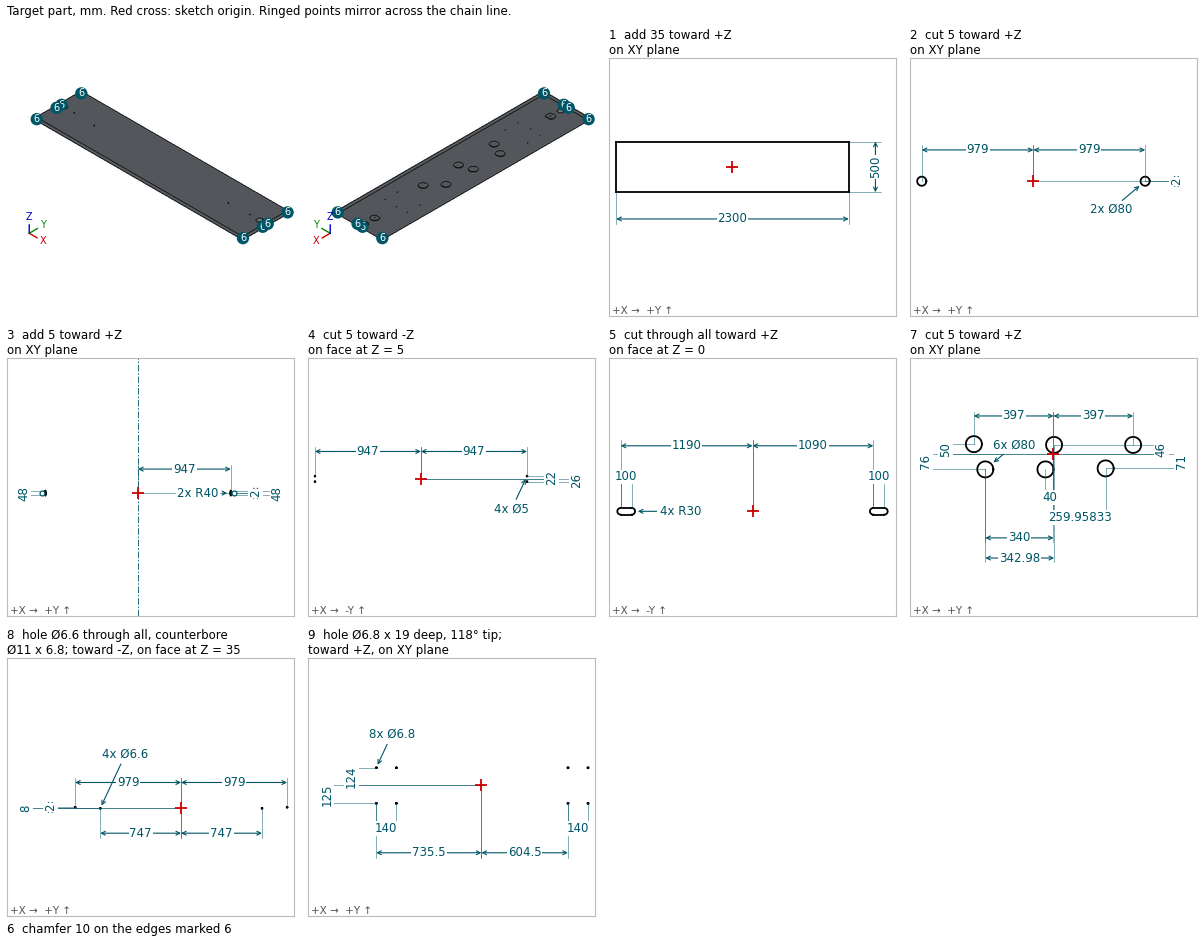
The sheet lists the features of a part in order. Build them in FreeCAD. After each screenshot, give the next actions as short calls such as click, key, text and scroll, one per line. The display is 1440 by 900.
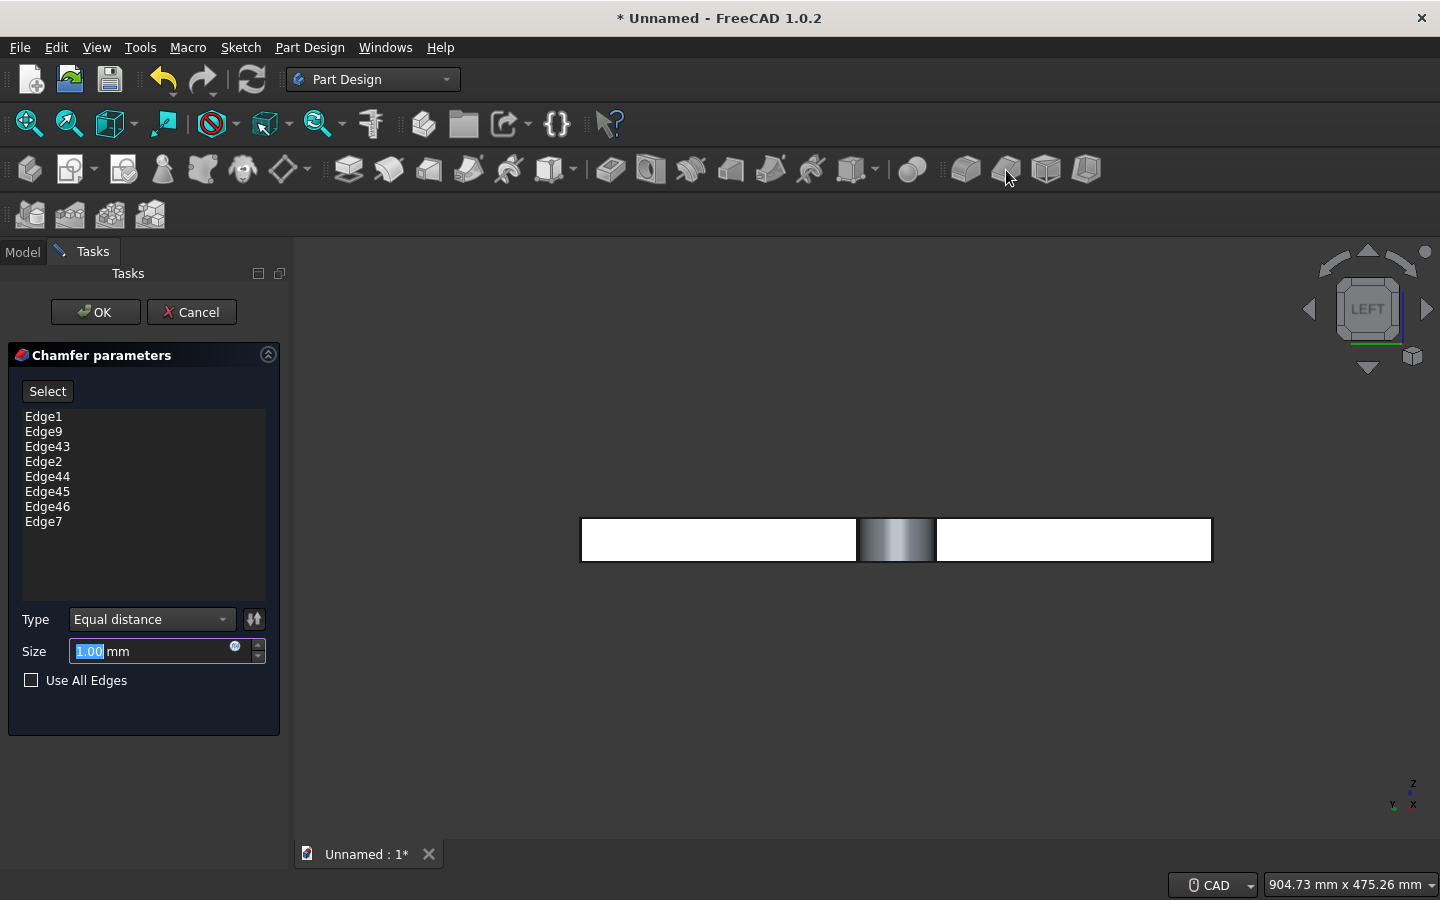
text(10)
key(Tab)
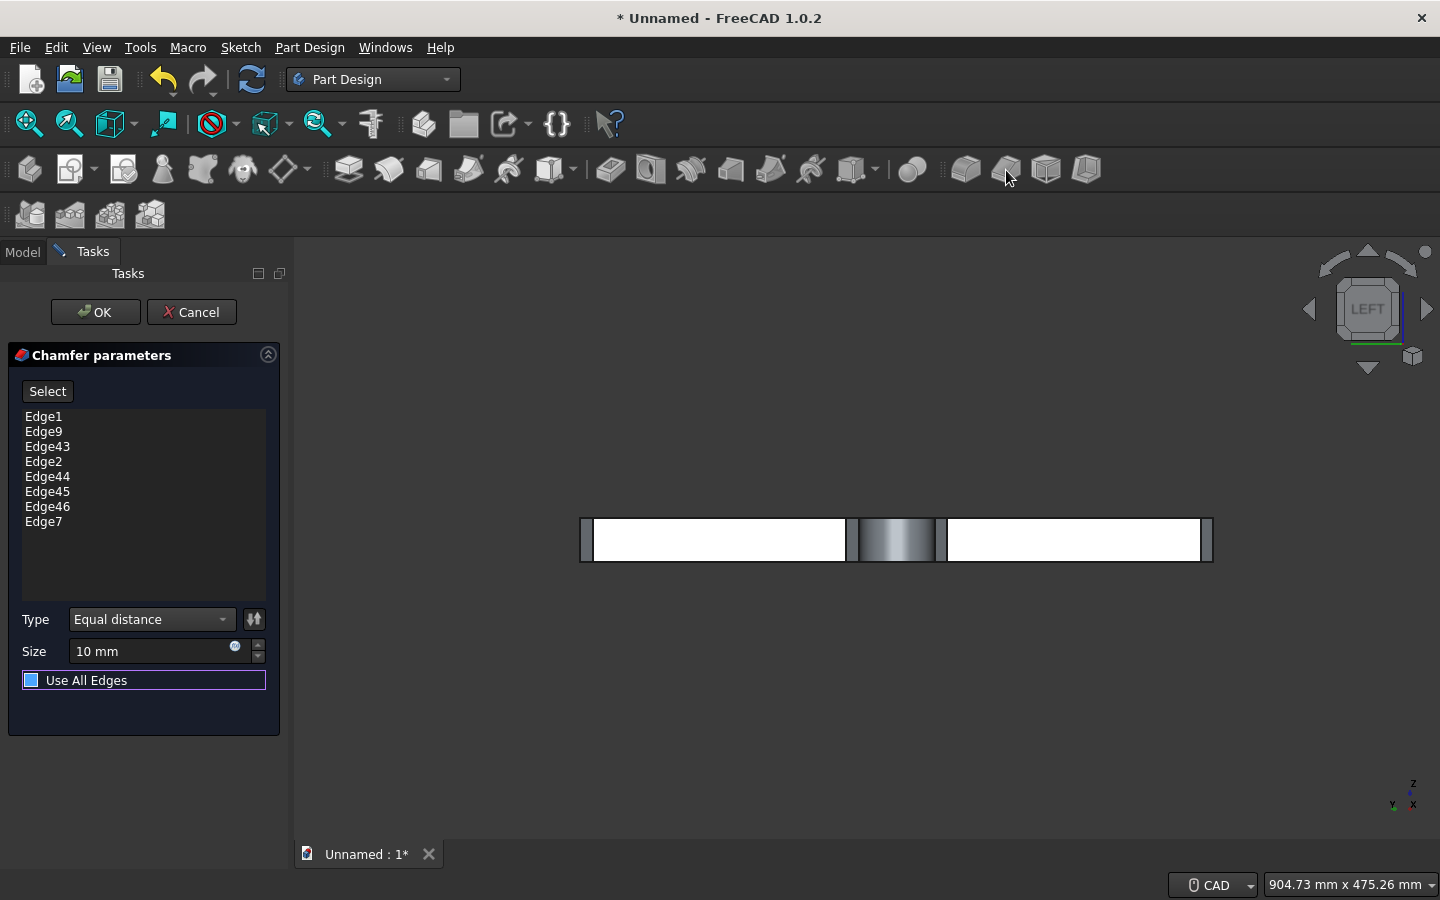
click(96, 312)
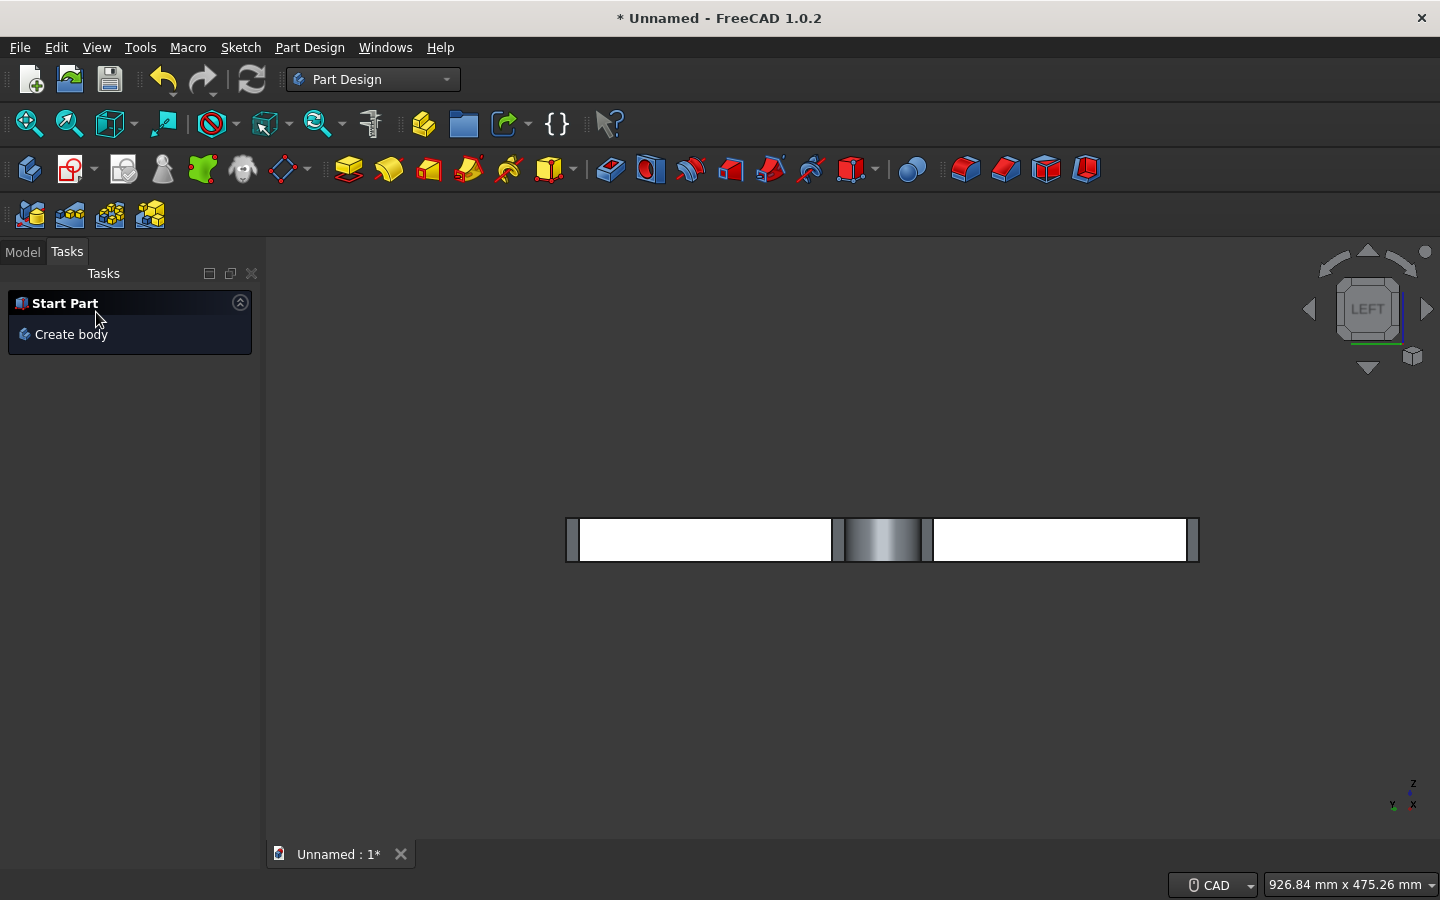
click(70, 170)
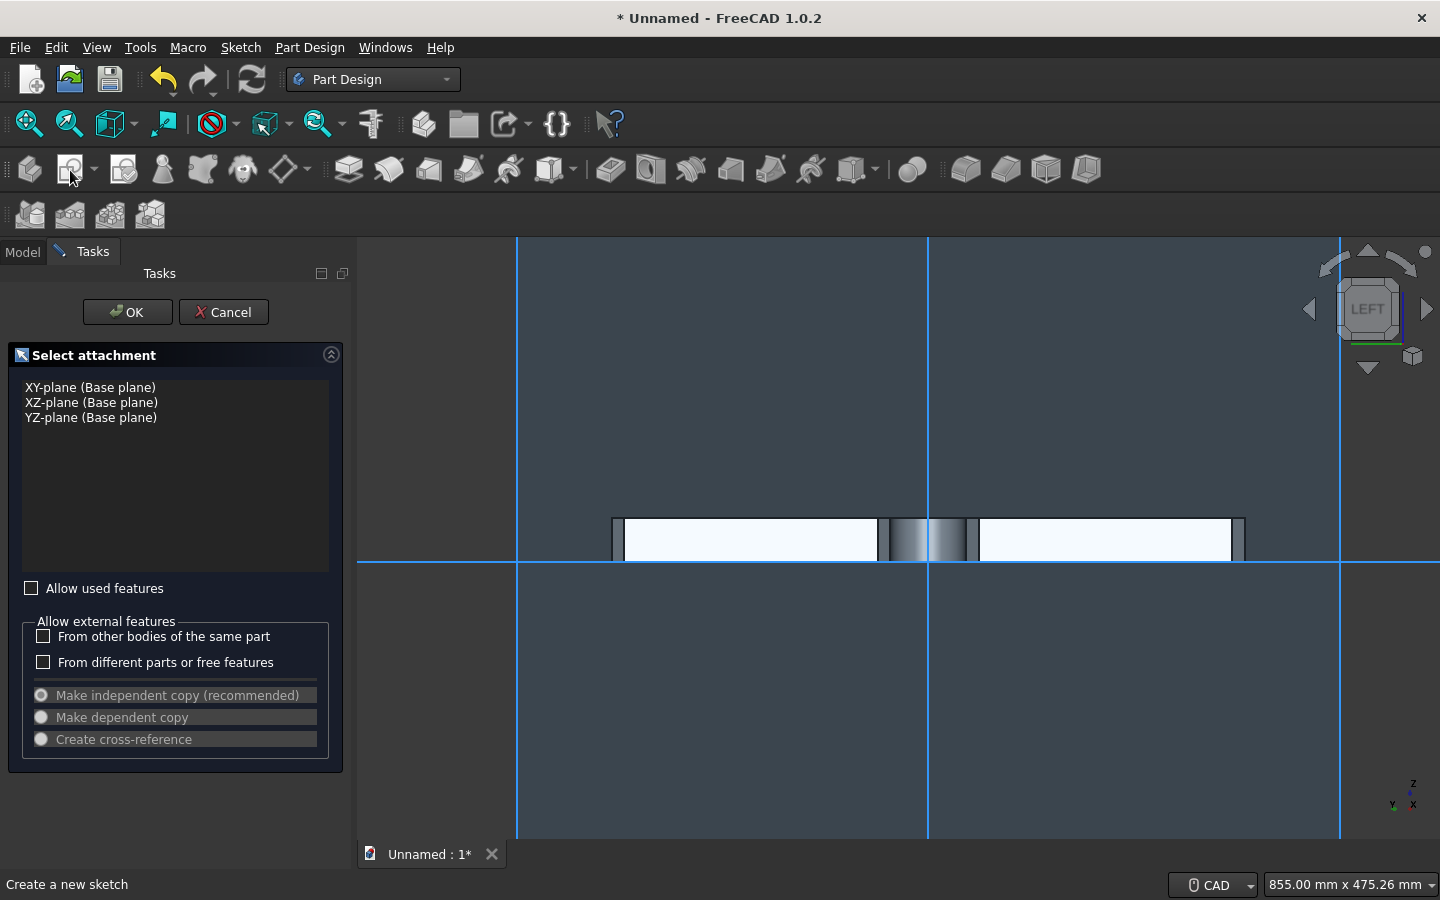
click(82, 388)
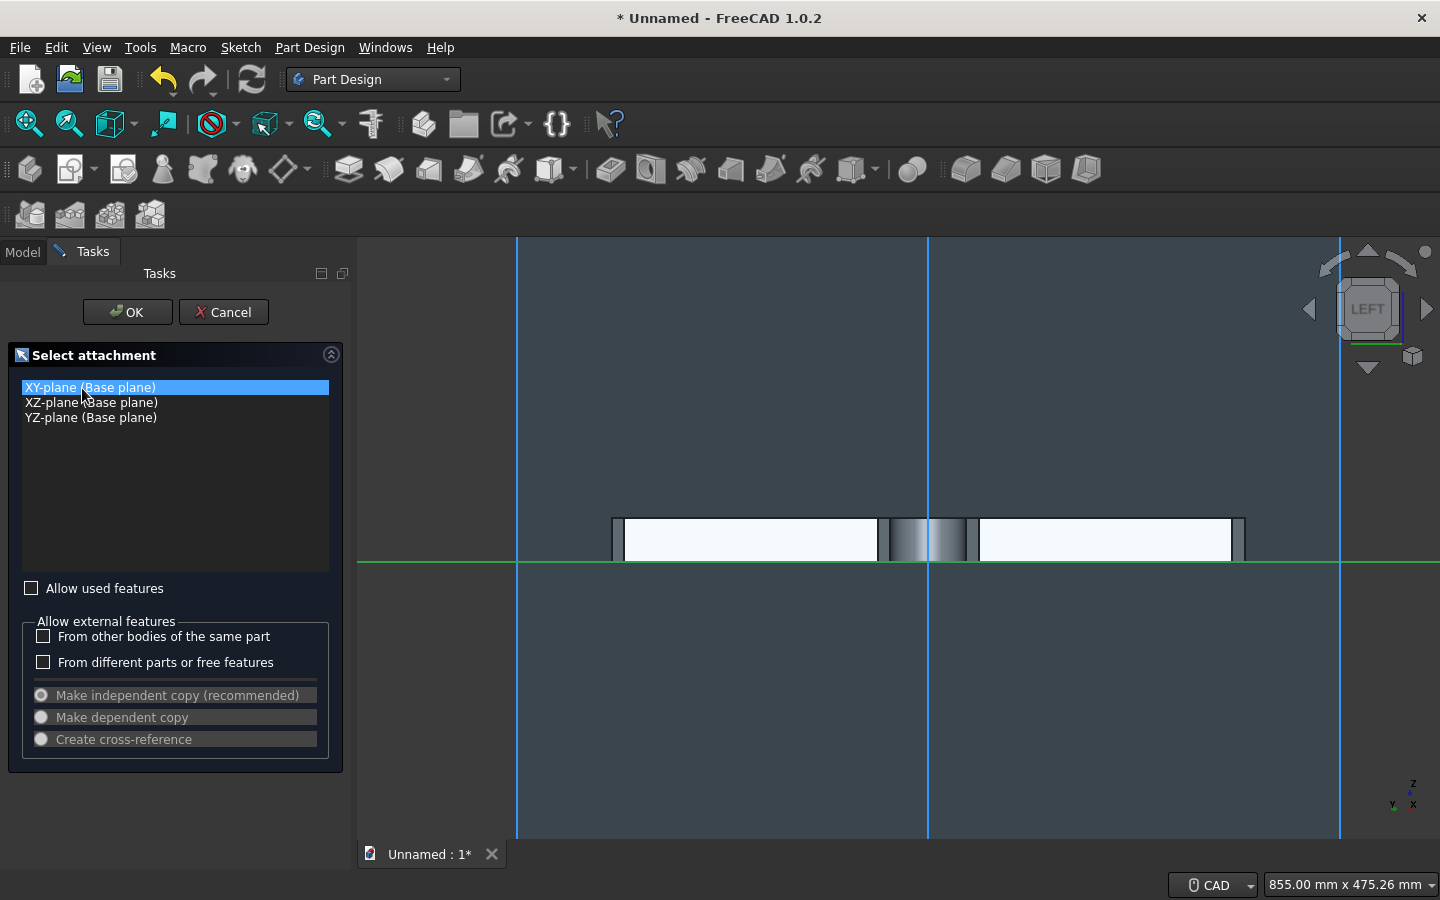
click(128, 312)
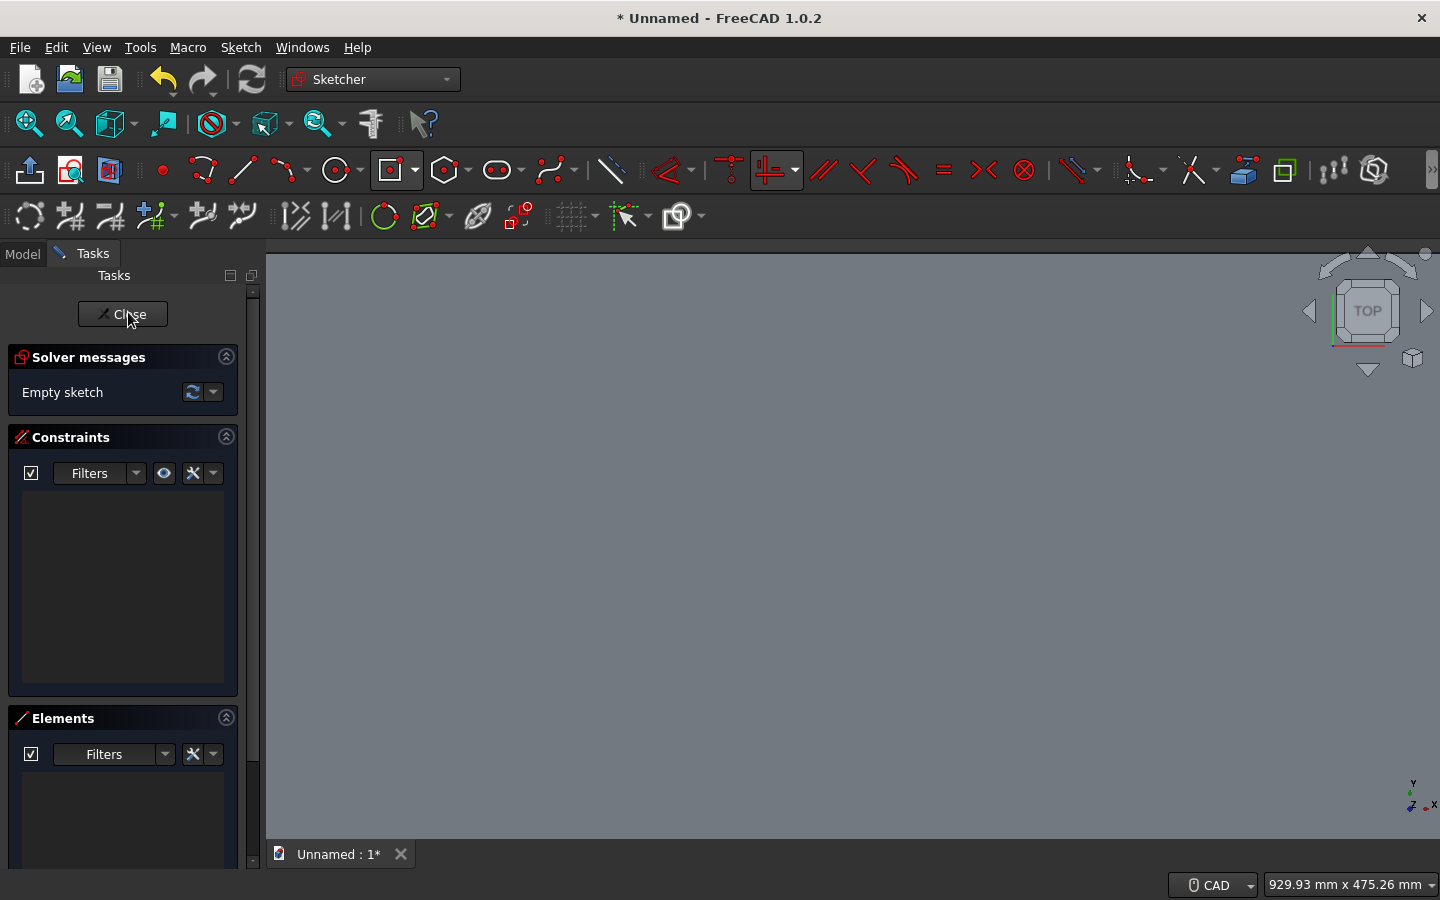
key(q)
key(s)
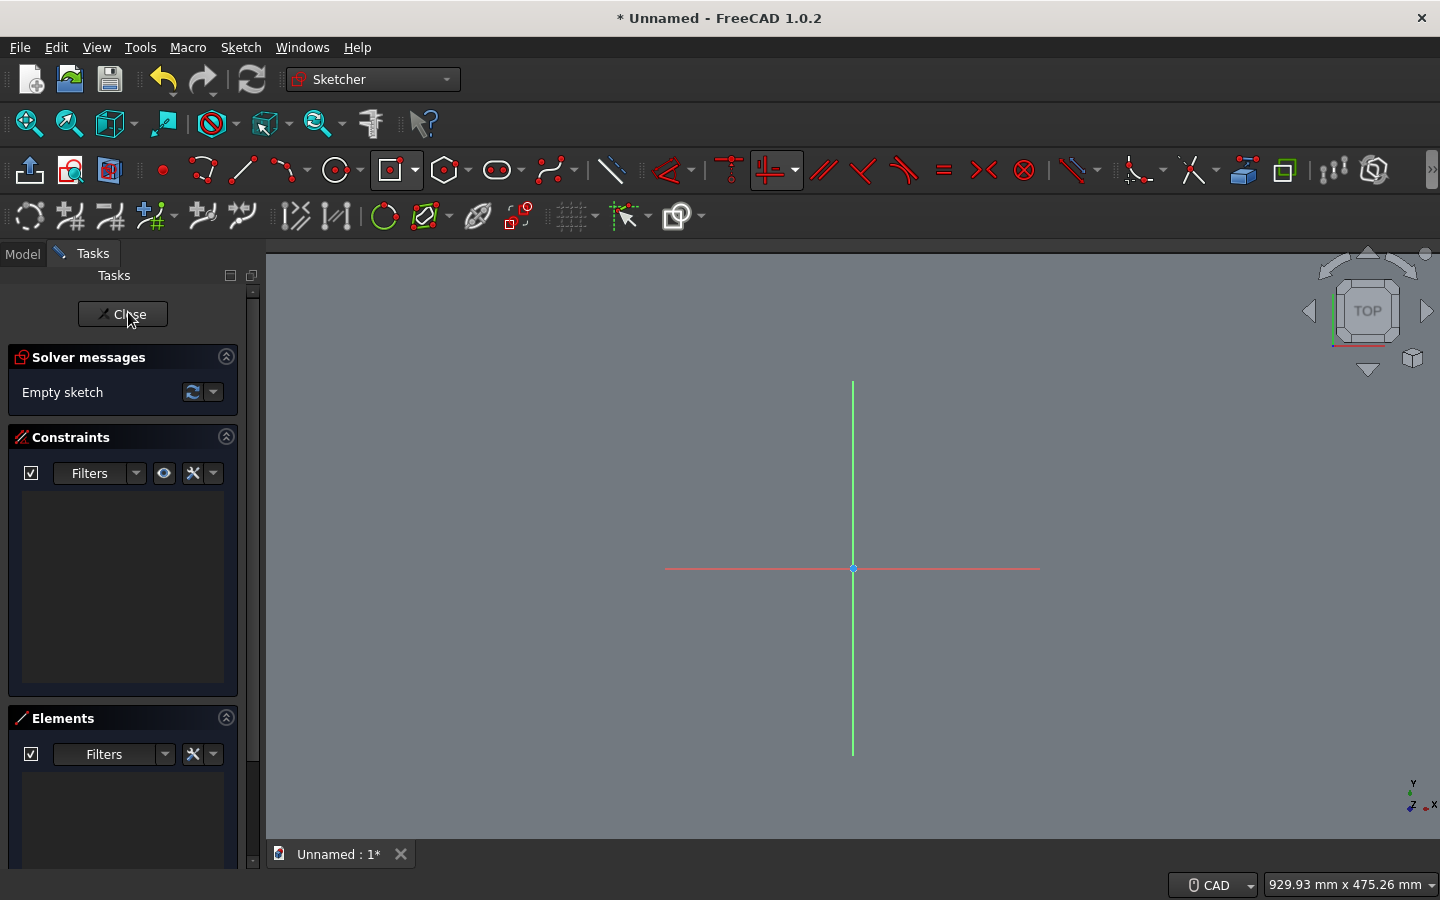
scroll(645, 445, down, 2)